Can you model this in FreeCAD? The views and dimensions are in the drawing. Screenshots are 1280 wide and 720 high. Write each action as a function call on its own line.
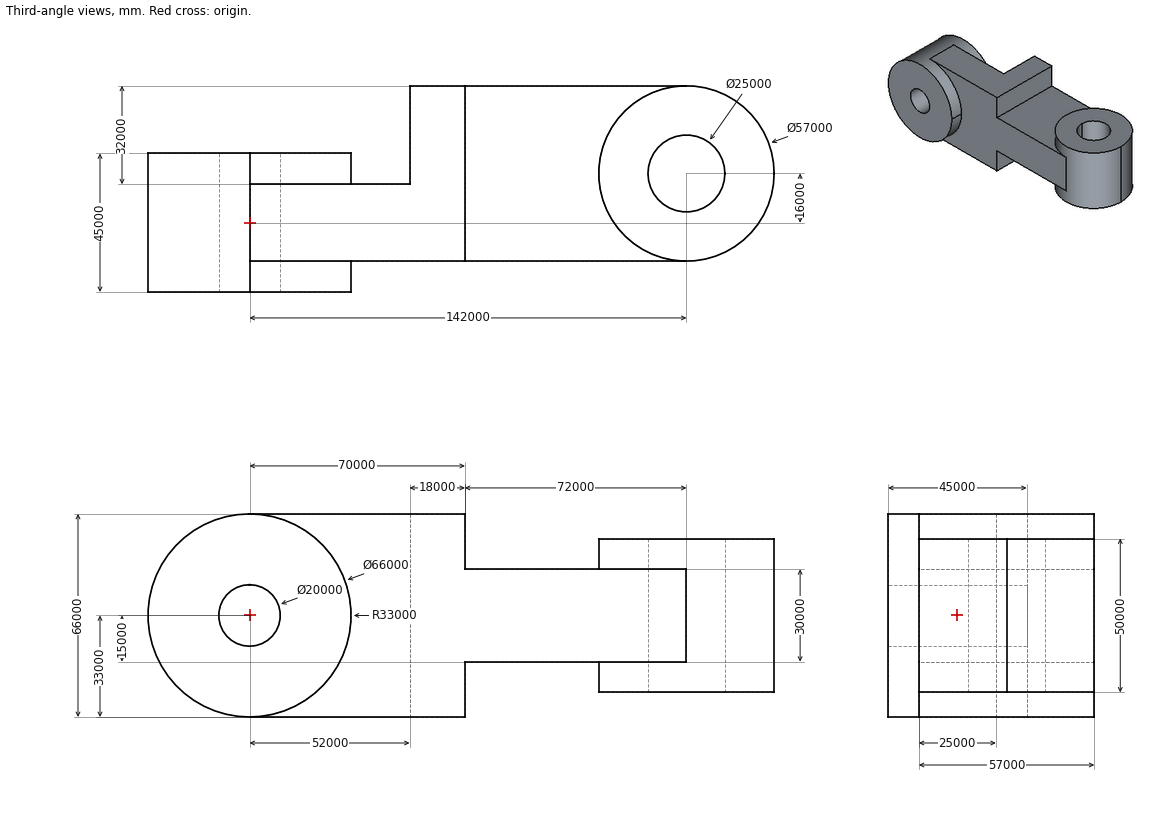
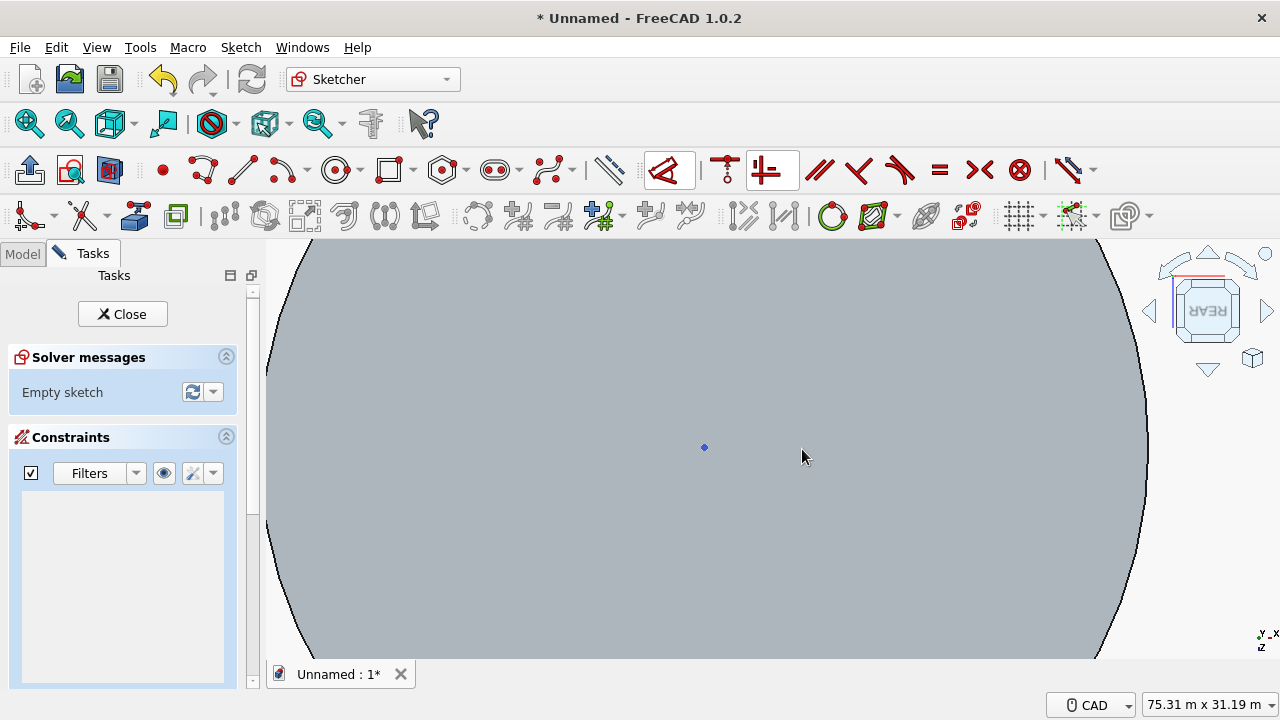
click(336, 170)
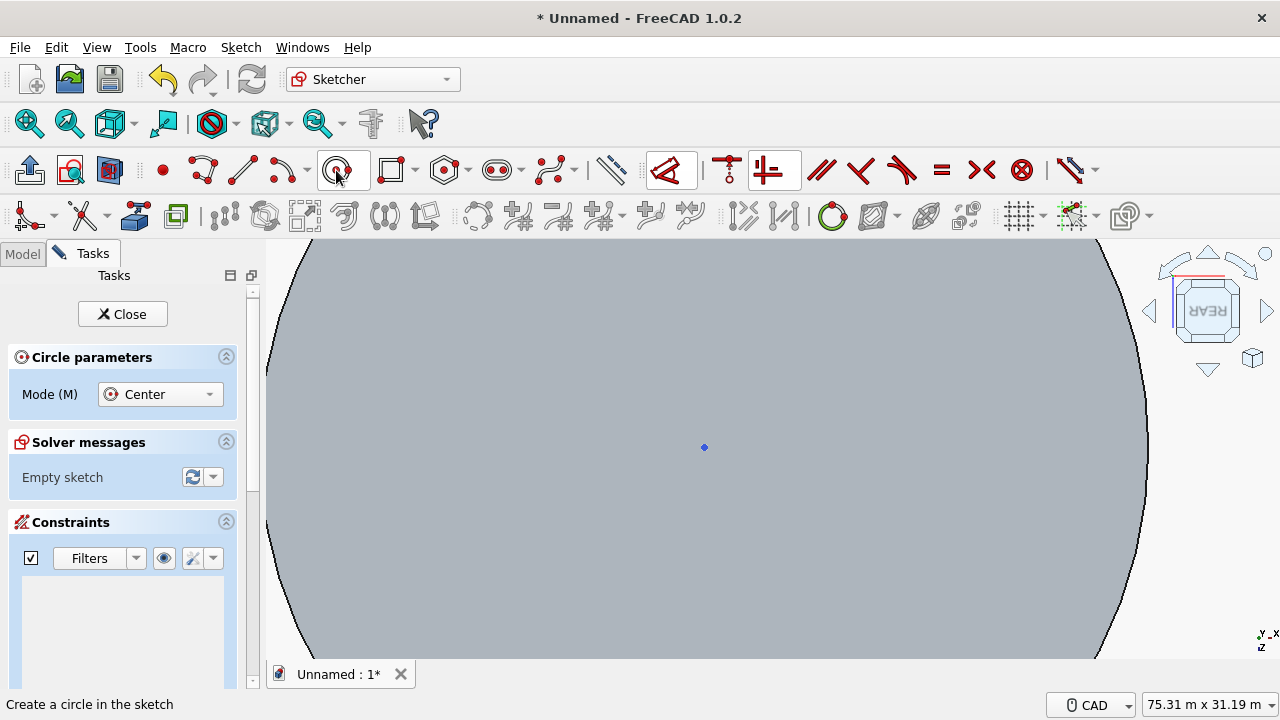
click(704, 448)
click(799, 353)
key(Escape)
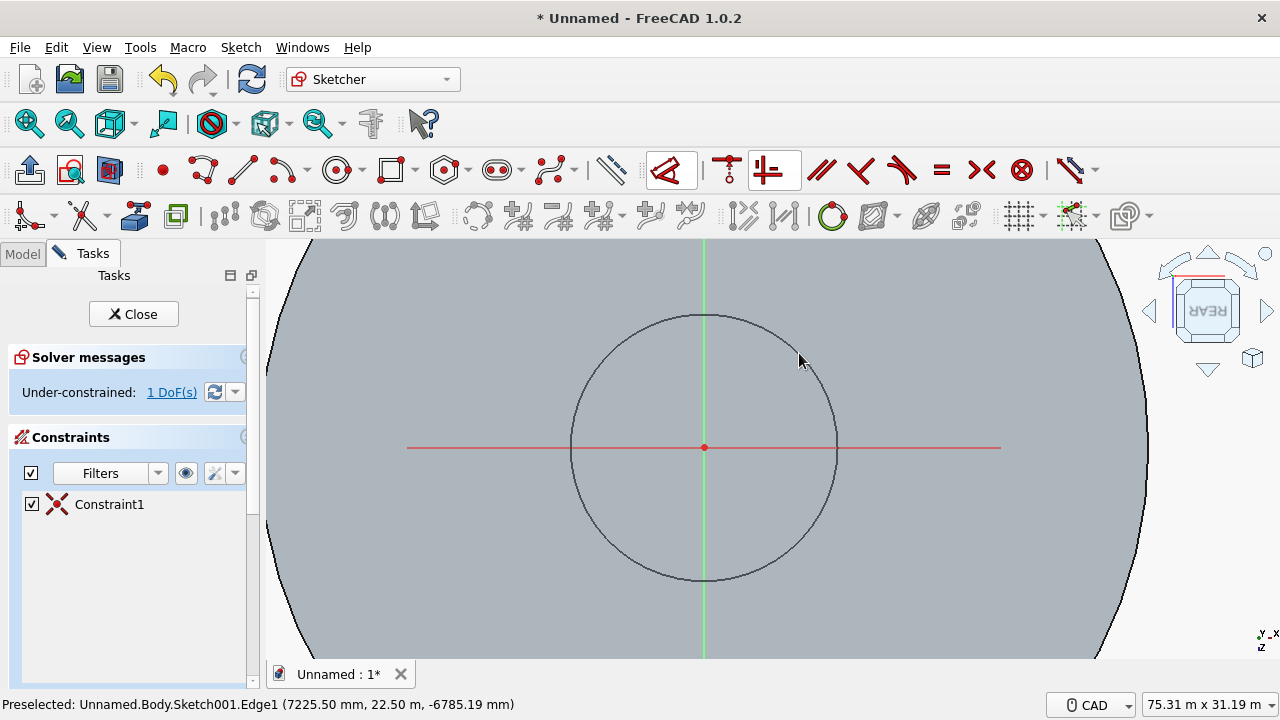
key(d)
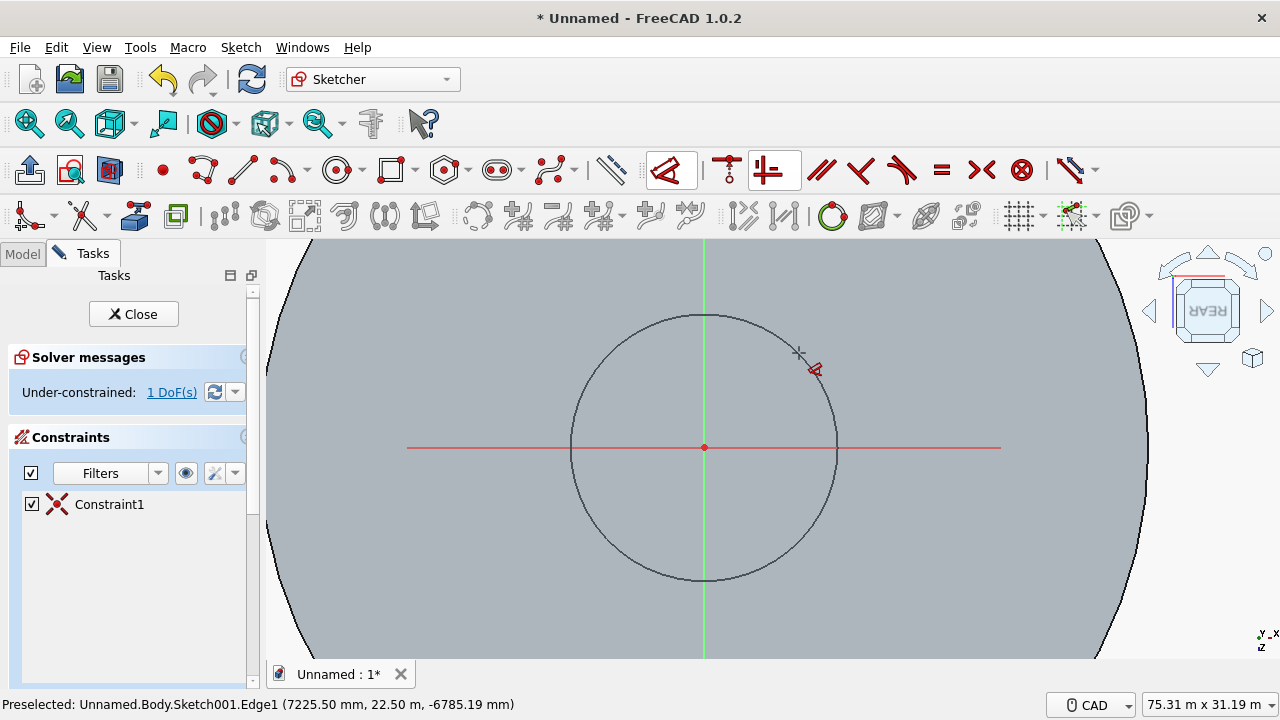
click(798, 353)
click(821, 330)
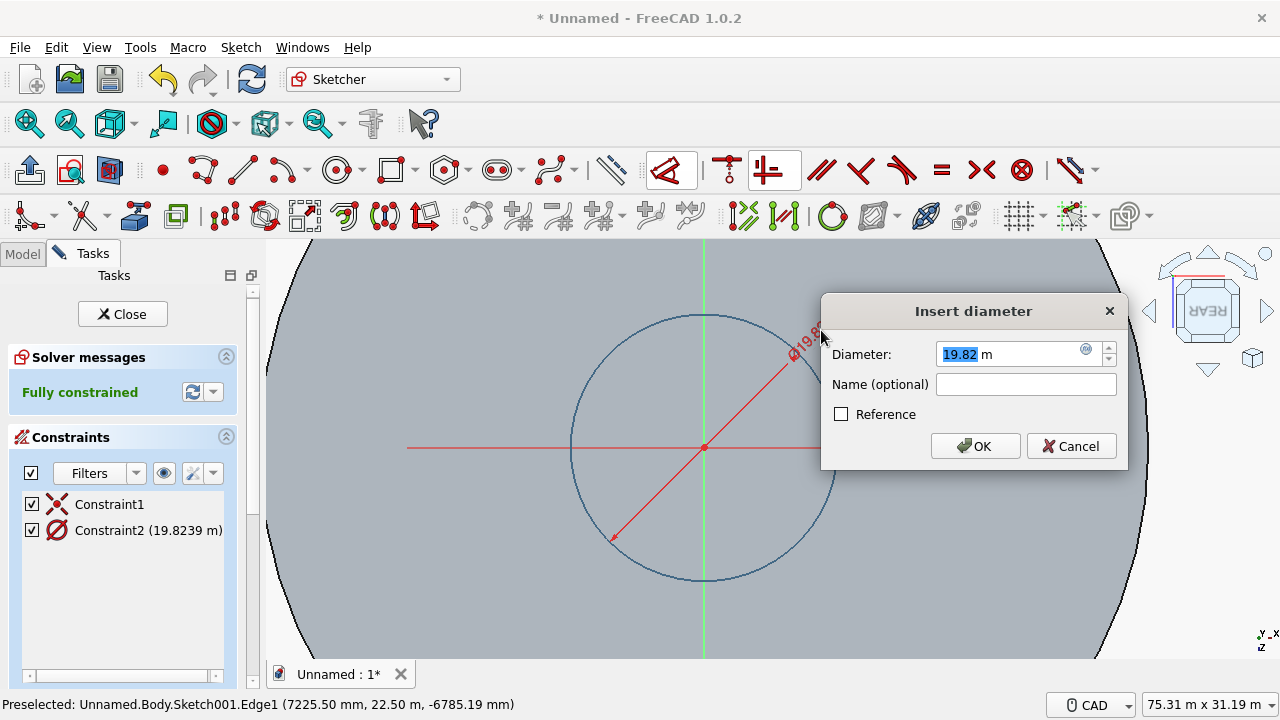
key(ctrl+a)
text(20000 mm)
key(Return)
key(Escape)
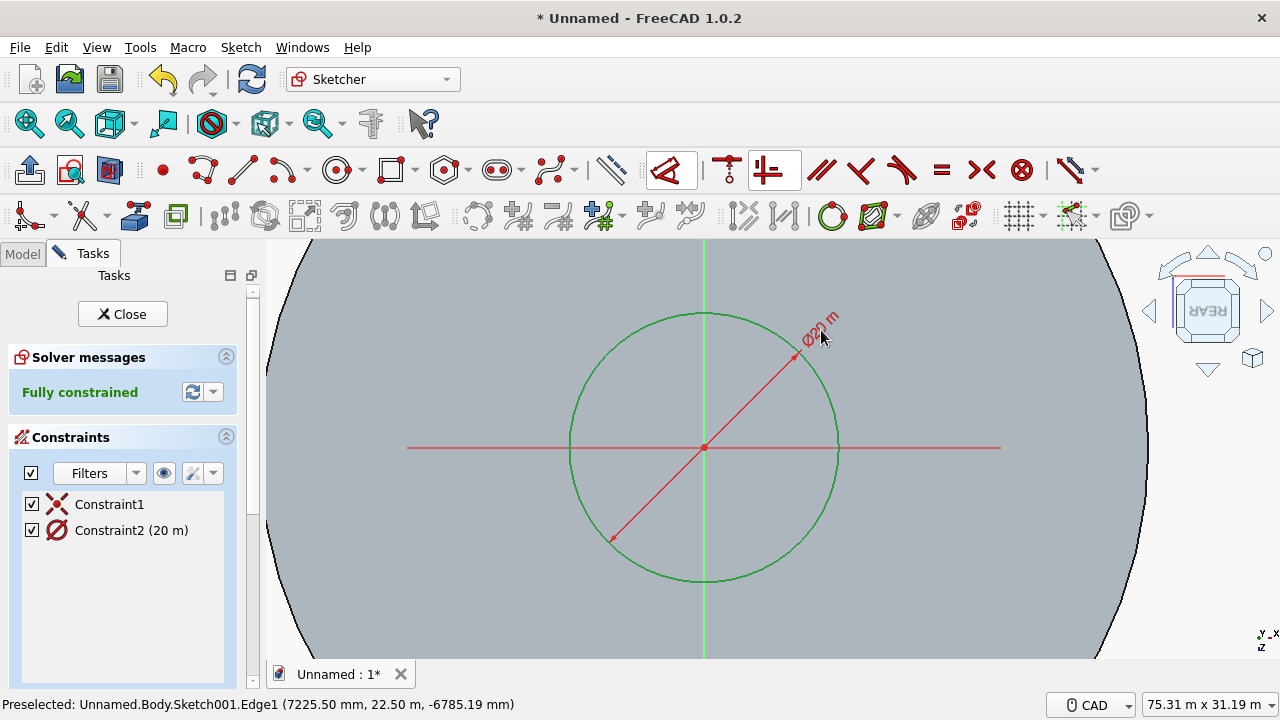
click(123, 314)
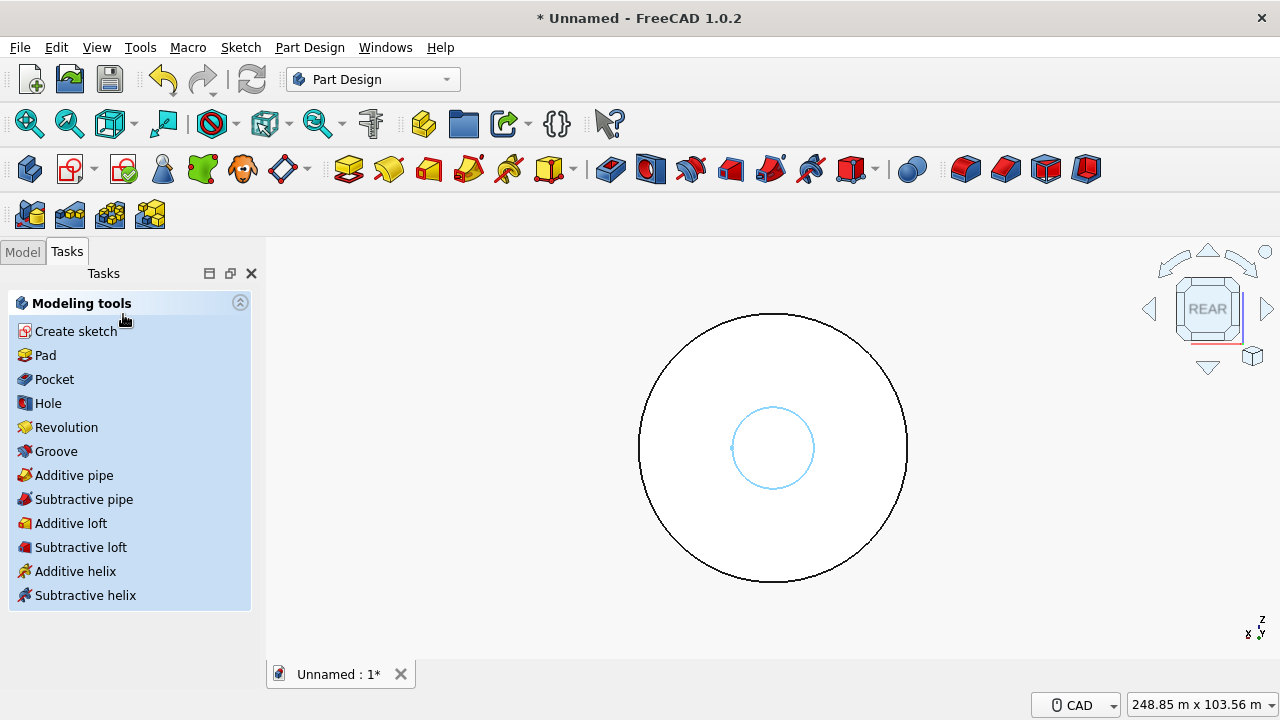
click(612, 170)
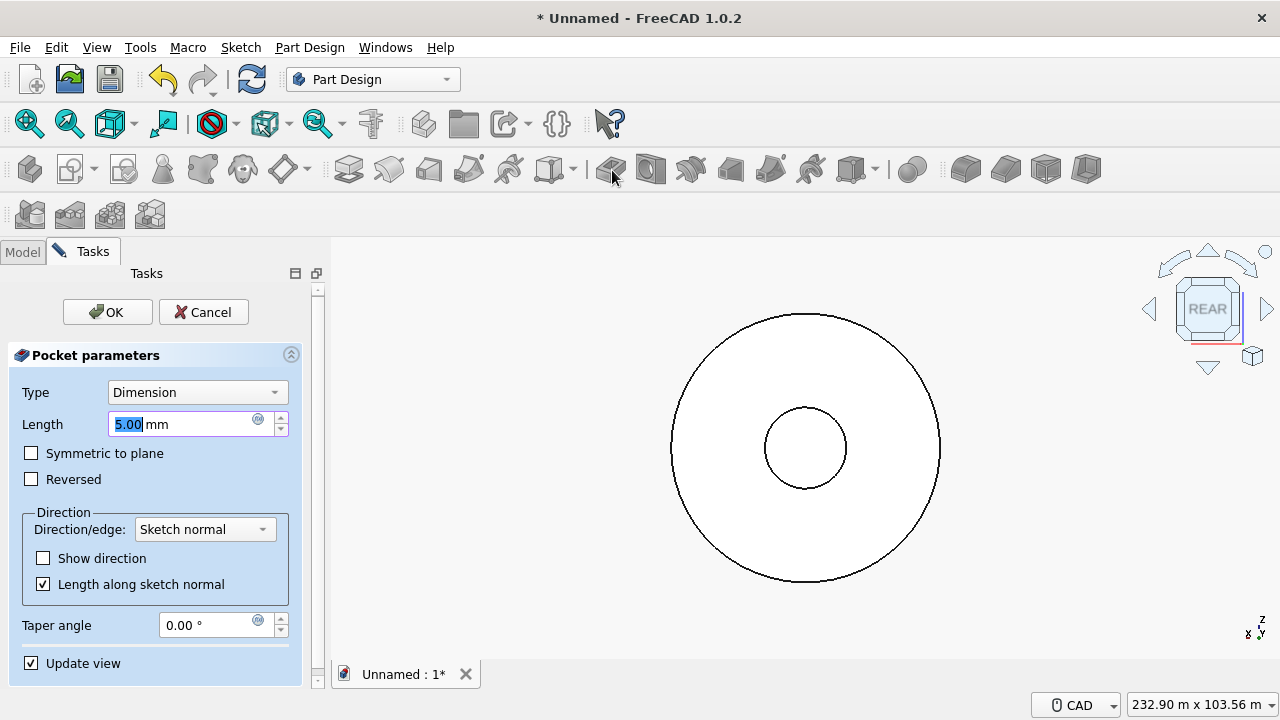
text(45000)
key(Tab)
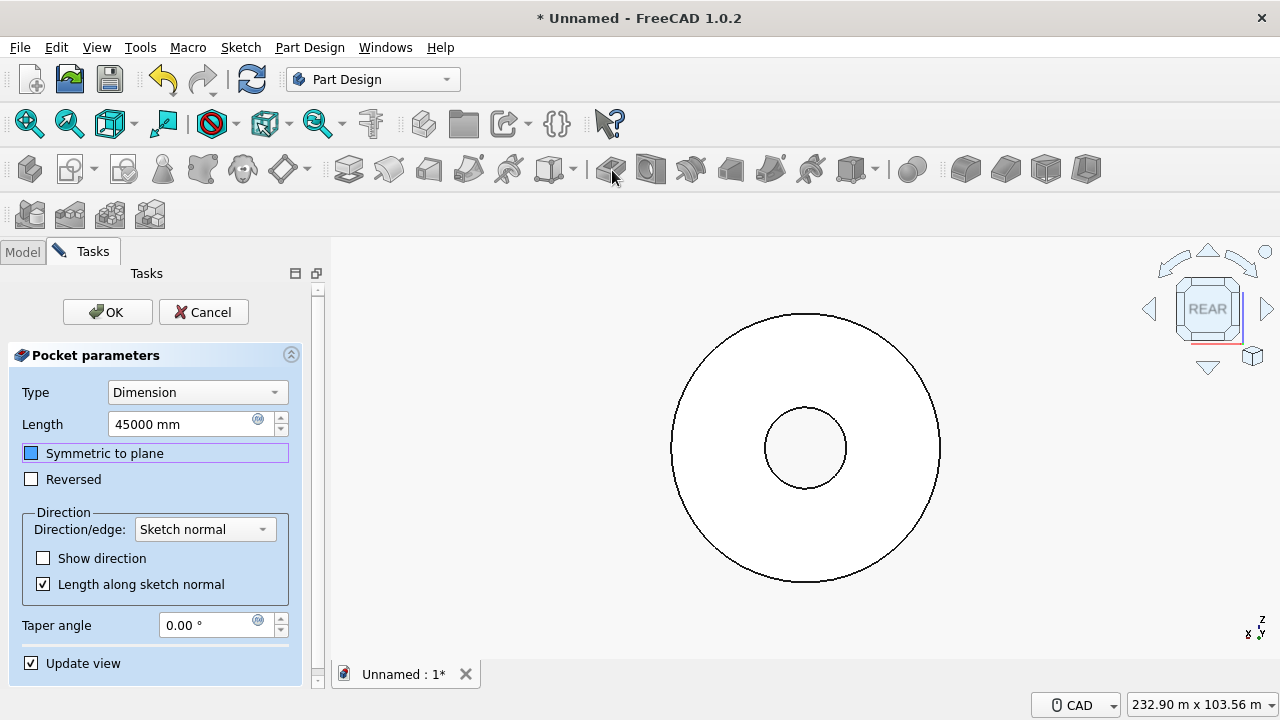
click(108, 312)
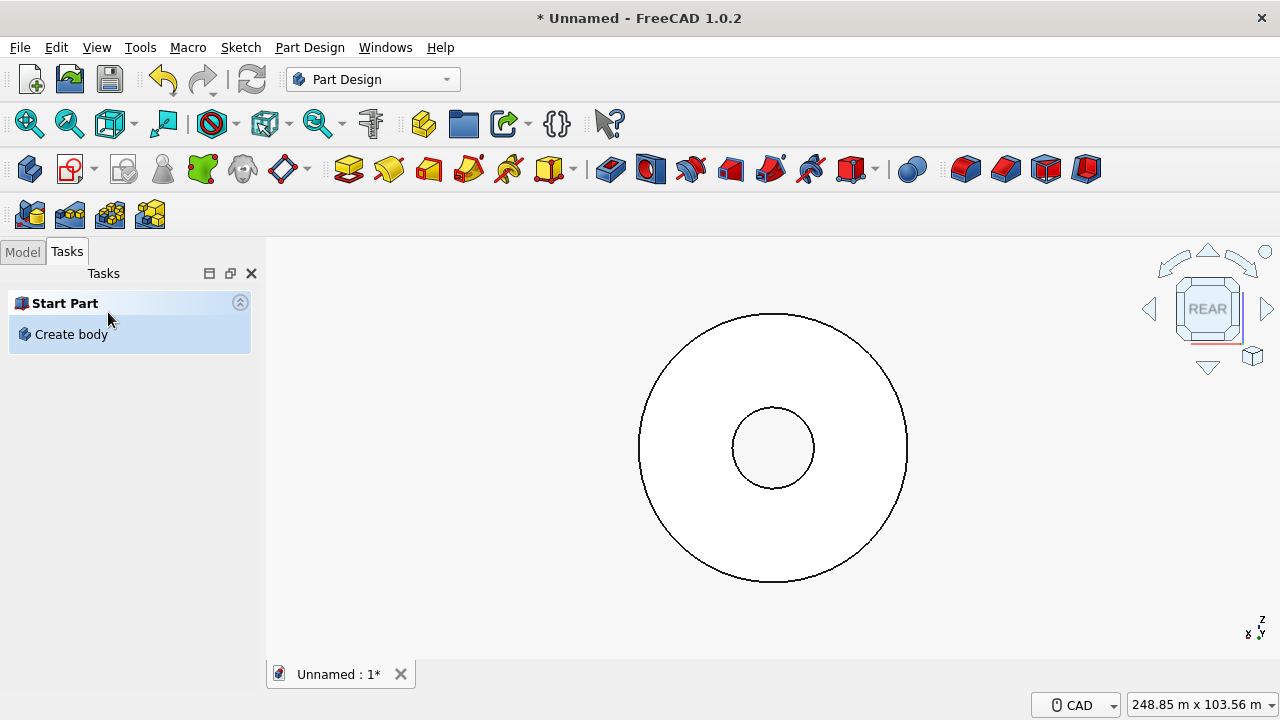
click(70, 170)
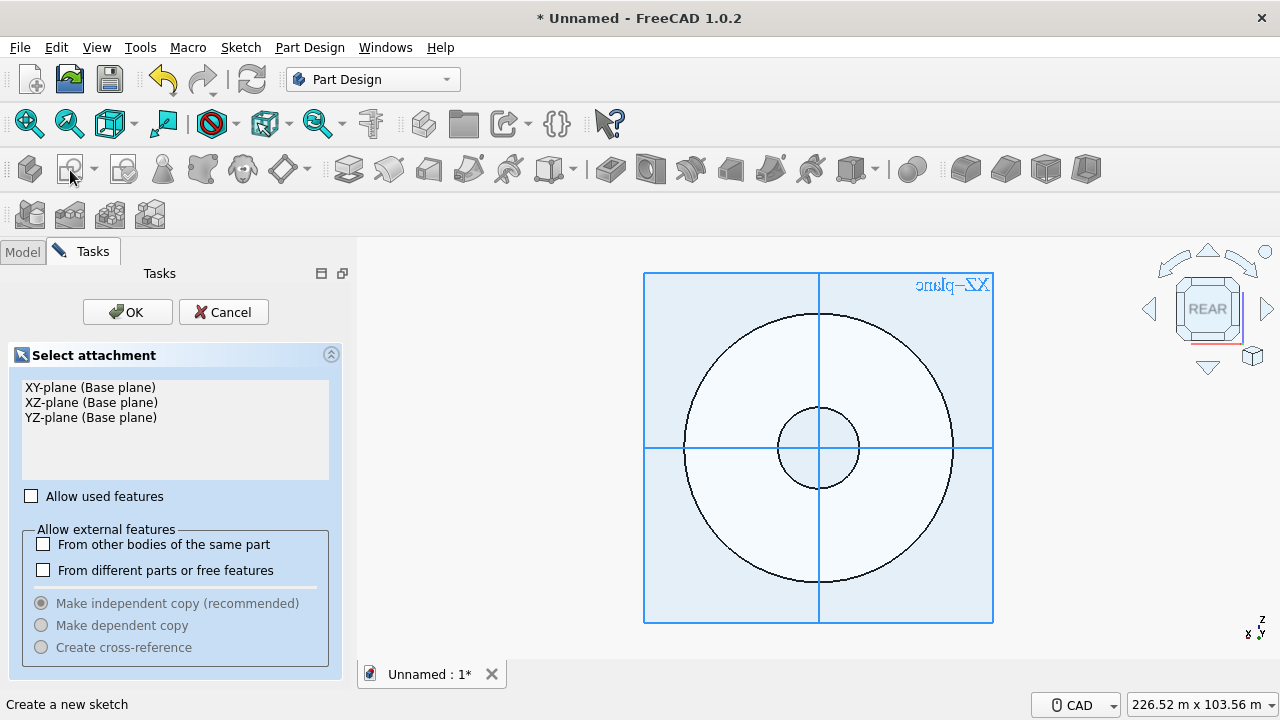
click(82, 402)